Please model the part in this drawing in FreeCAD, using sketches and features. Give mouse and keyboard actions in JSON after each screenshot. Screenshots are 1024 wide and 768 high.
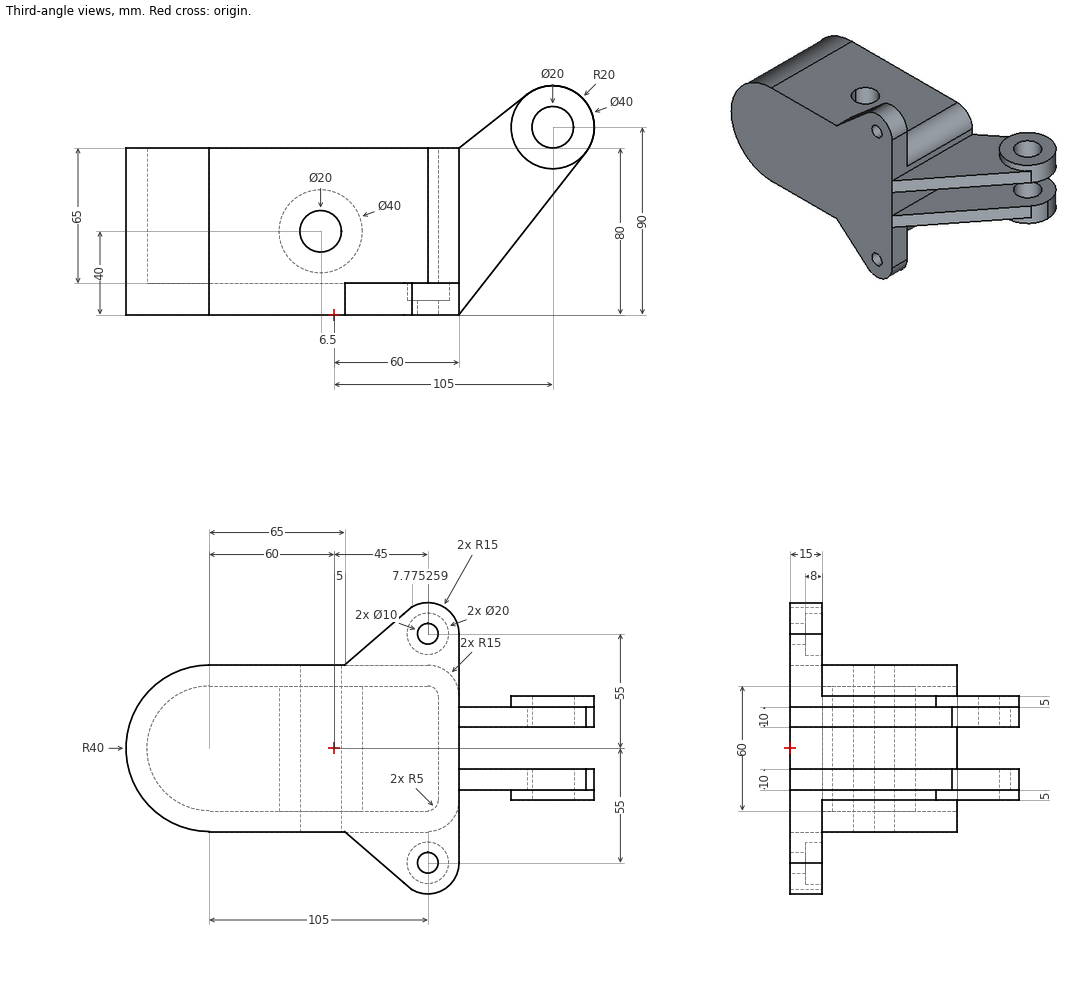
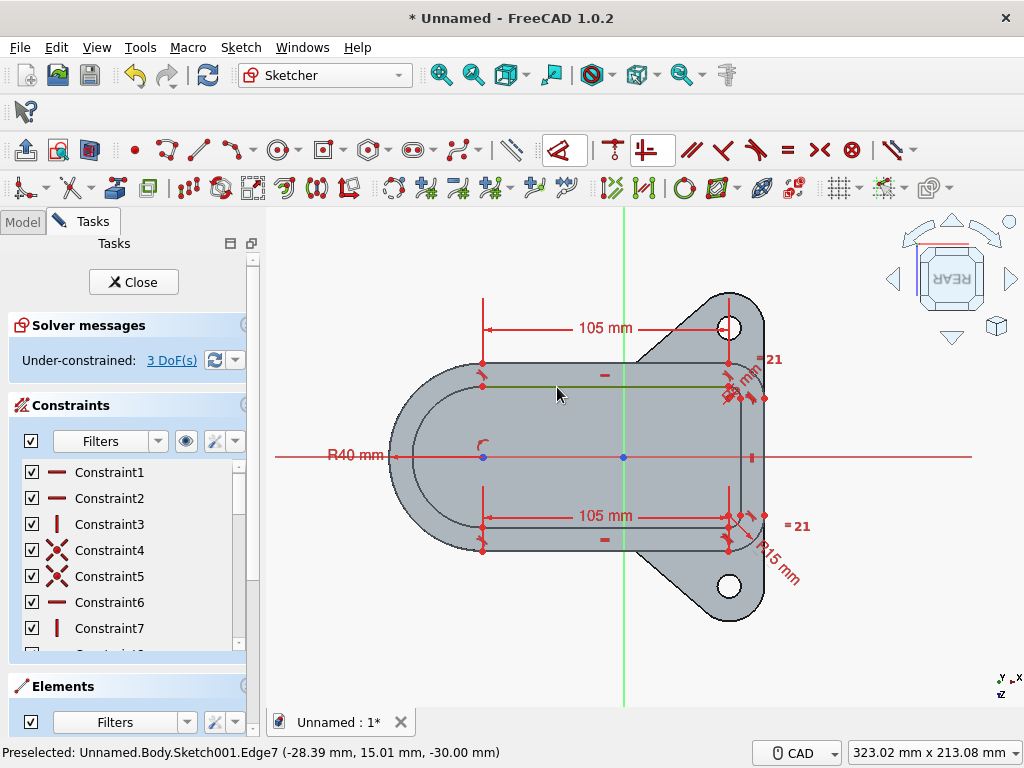
{"action": "key", "text": "l"}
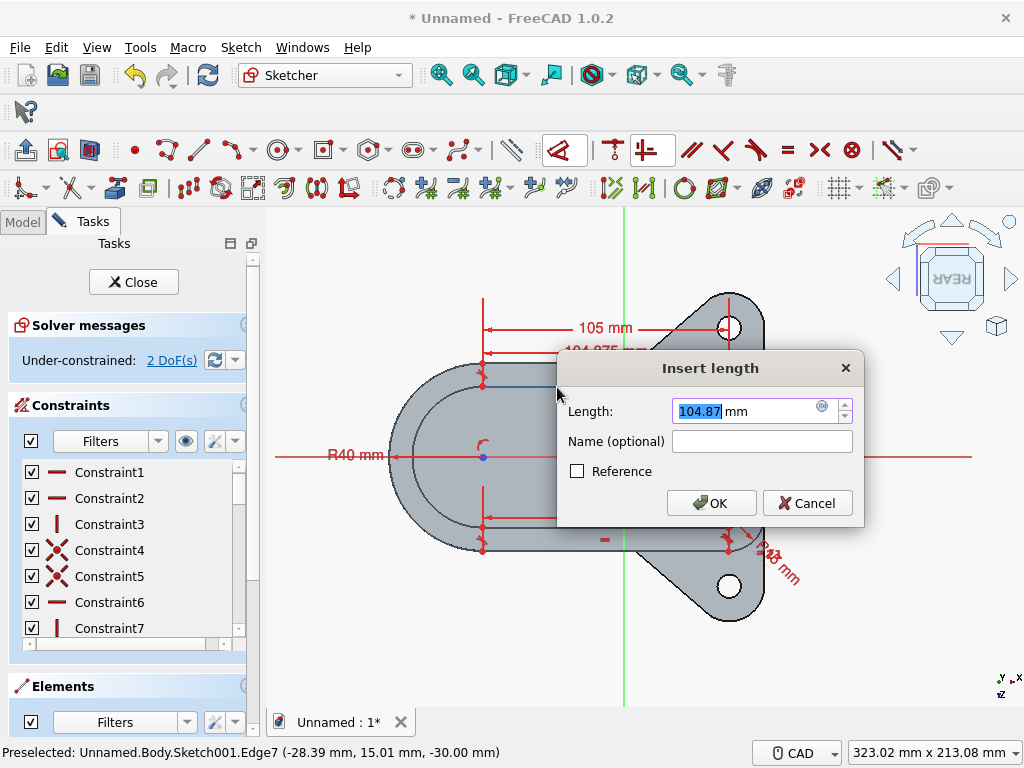
{"action": "type", "text": "105"}
{"action": "key", "text": "Return"}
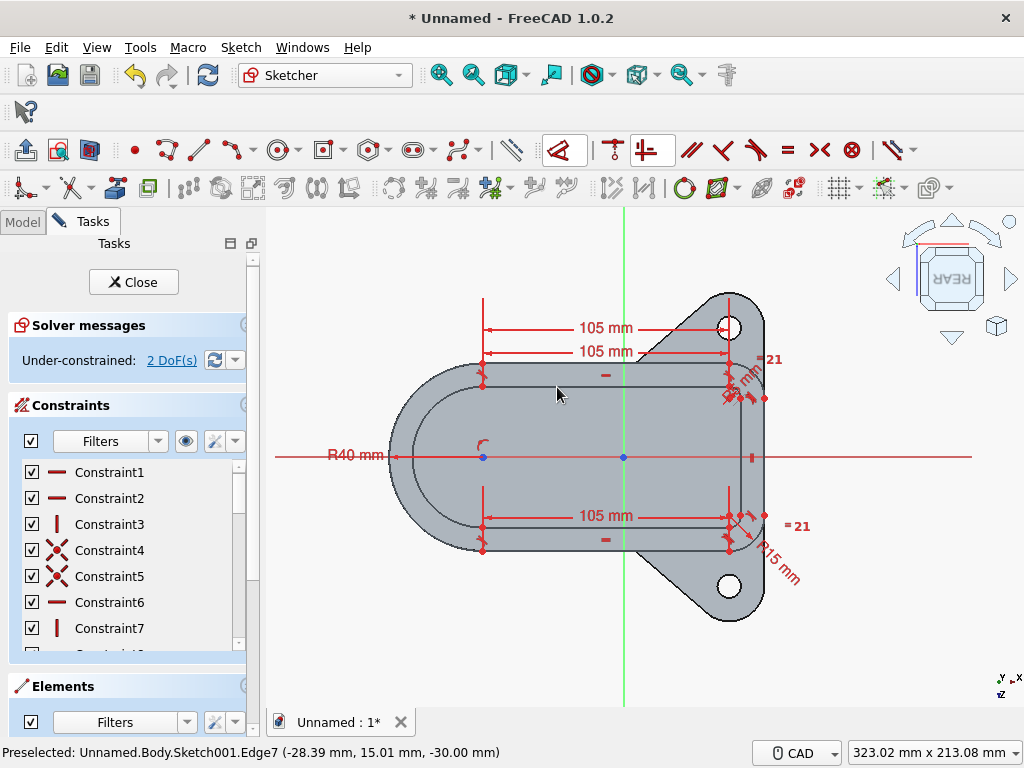
{"action": "left_click", "coordinate": [729, 363]}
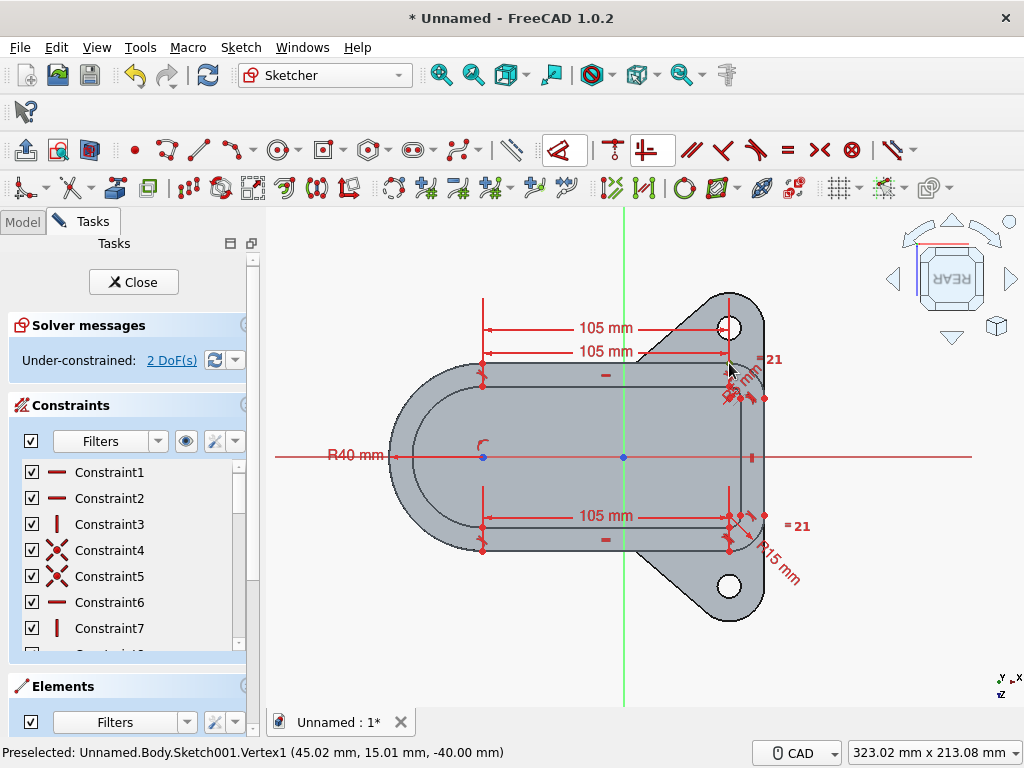
{"action": "left_click", "coordinate": [582, 150]}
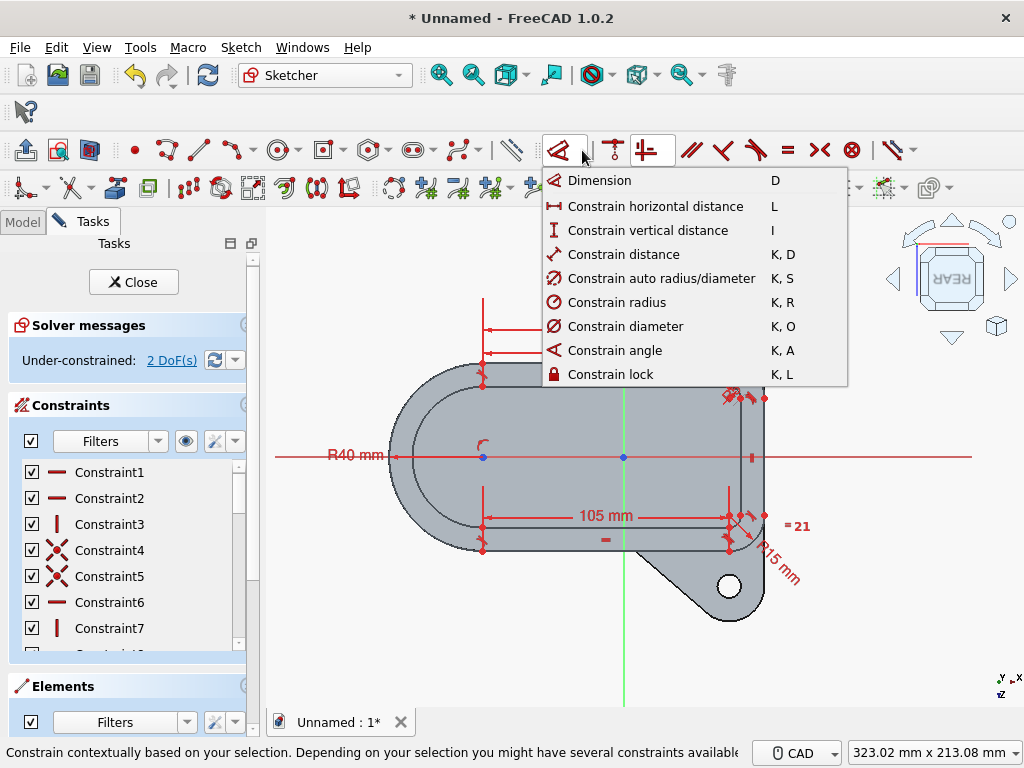
{"action": "left_click", "coordinate": [695, 206]}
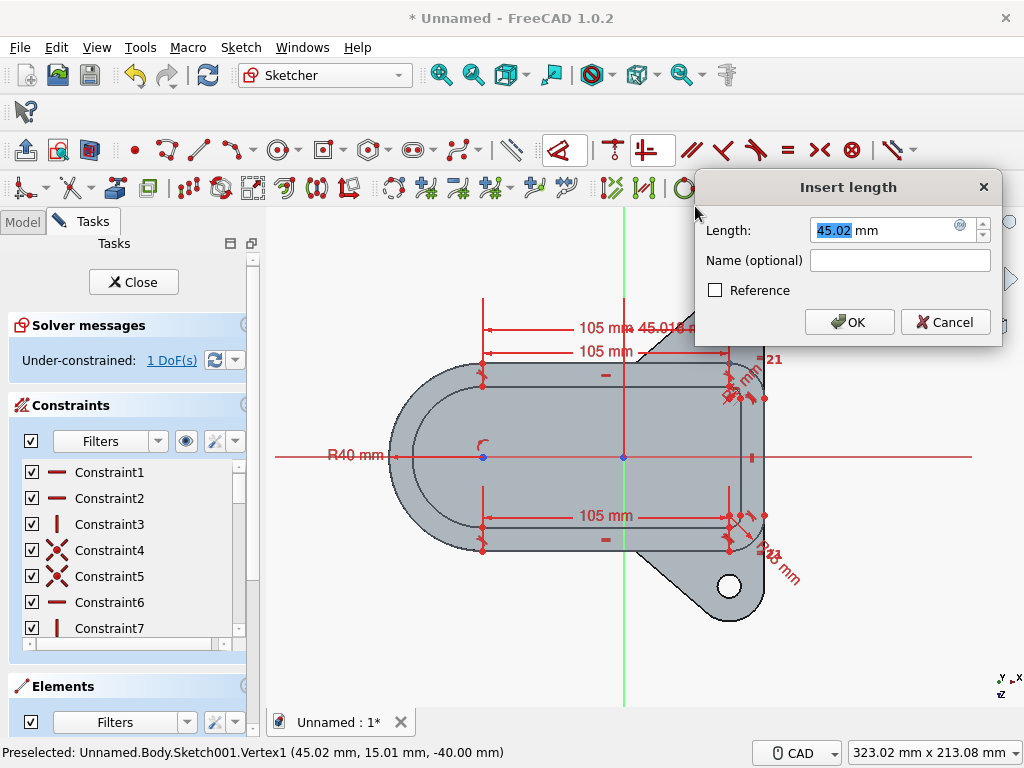
{"action": "type", "text": "45"}
{"action": "key", "text": "Return"}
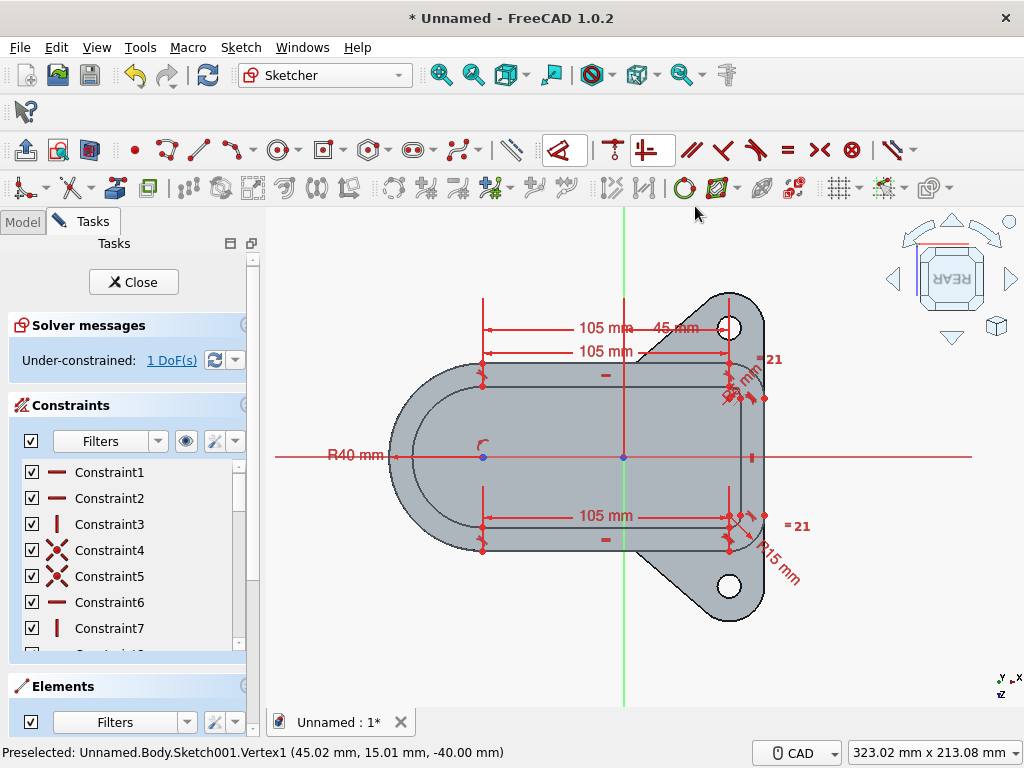
{"action": "left_click", "coordinate": [483, 457]}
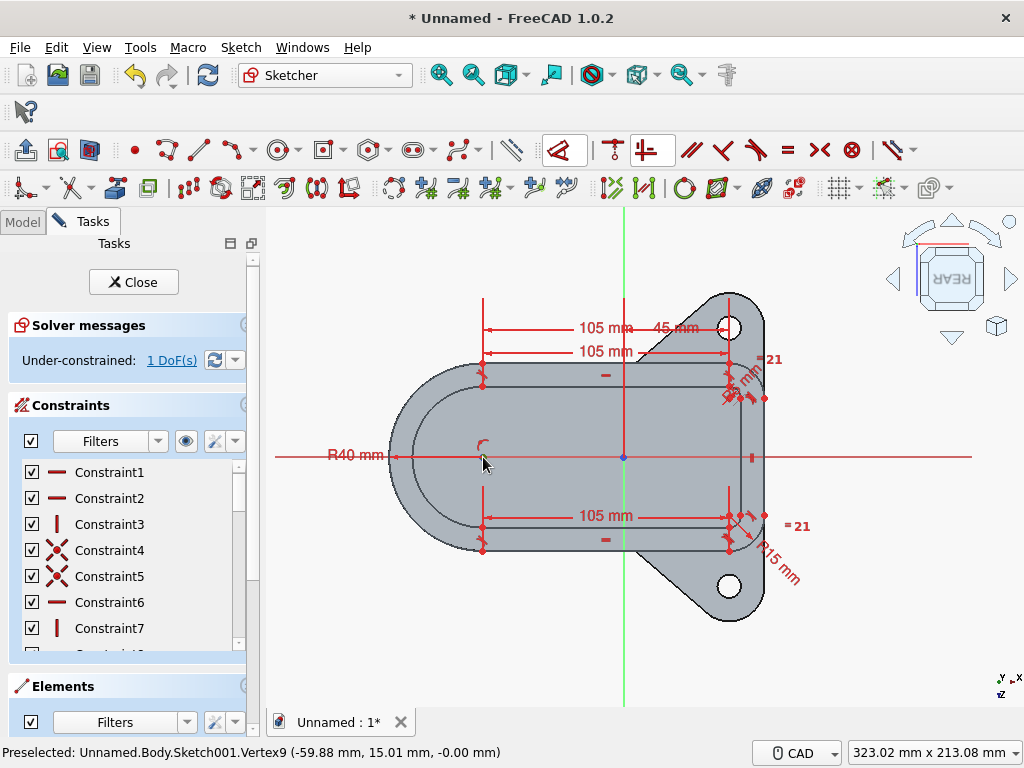
{"action": "key", "text": "l"}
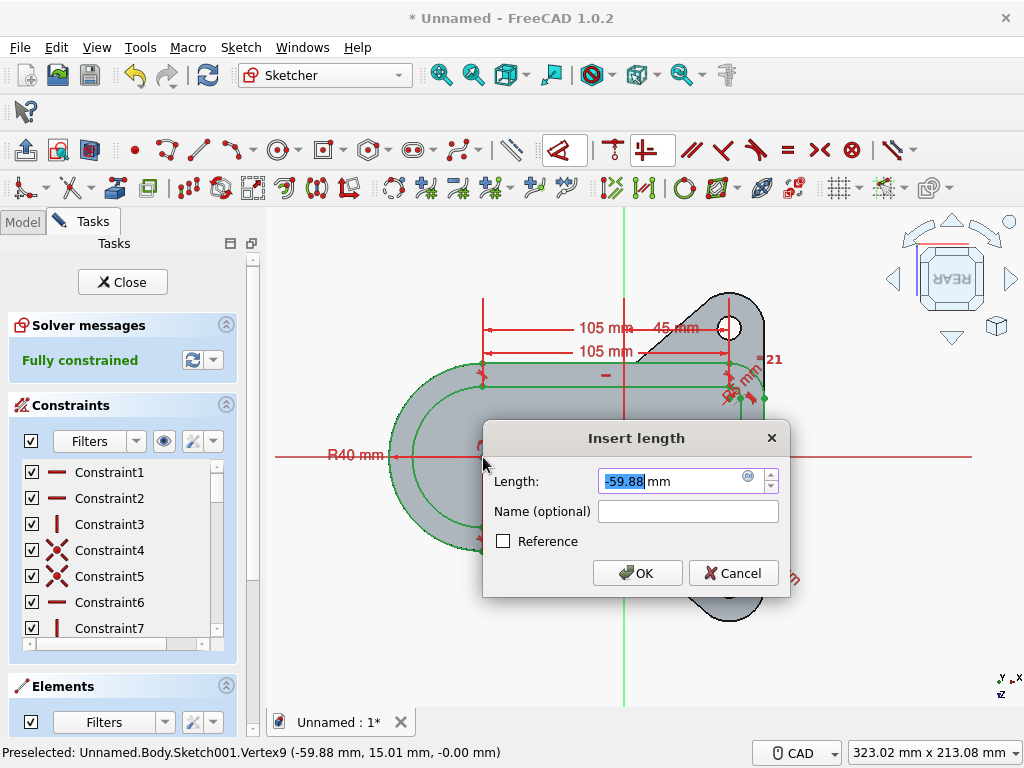
{"action": "type", "text": "-60"}
{"action": "key", "text": "Return"}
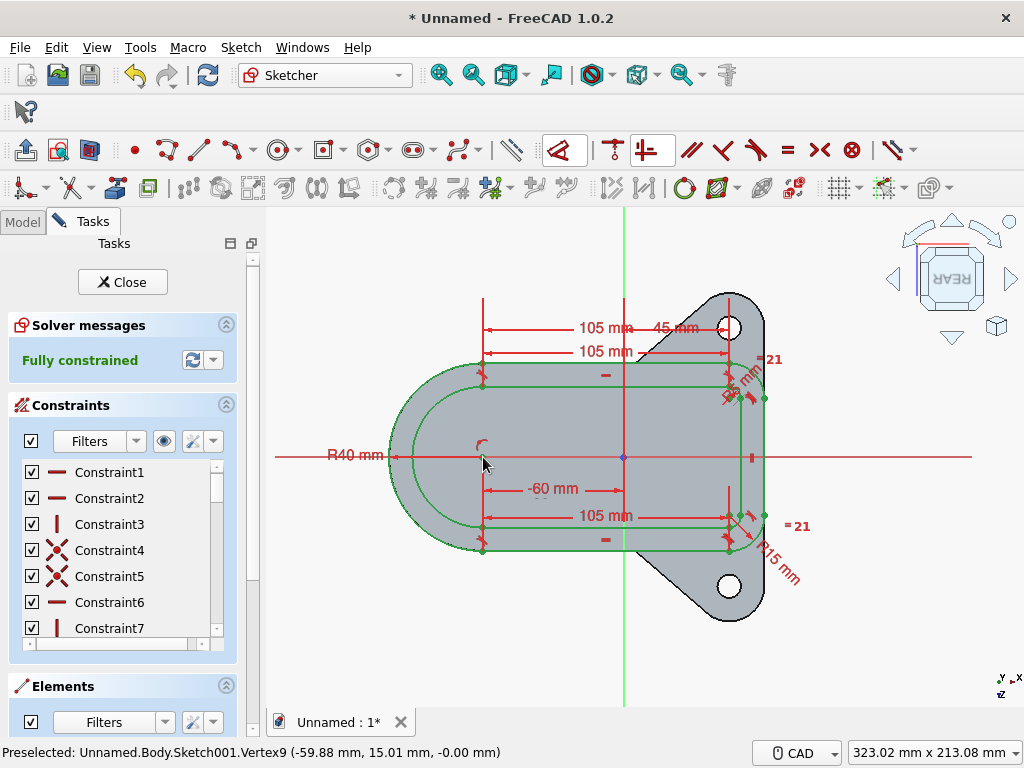
{"action": "left_click", "coordinate": [123, 282]}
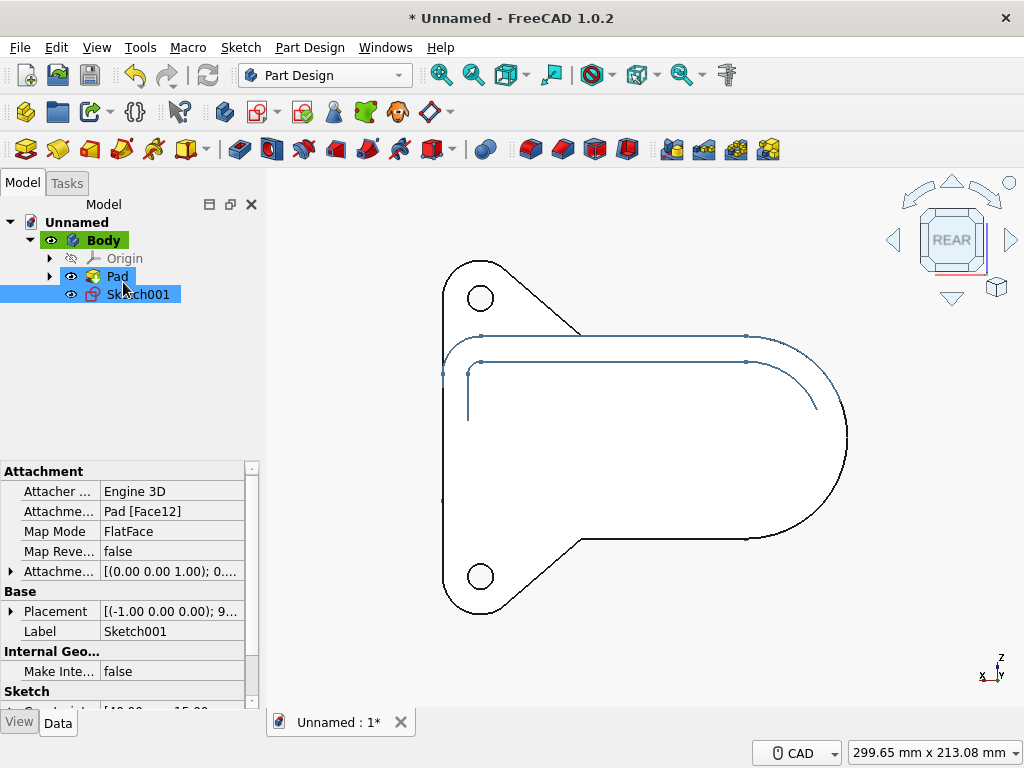
{"action": "left_click", "coordinate": [26, 150]}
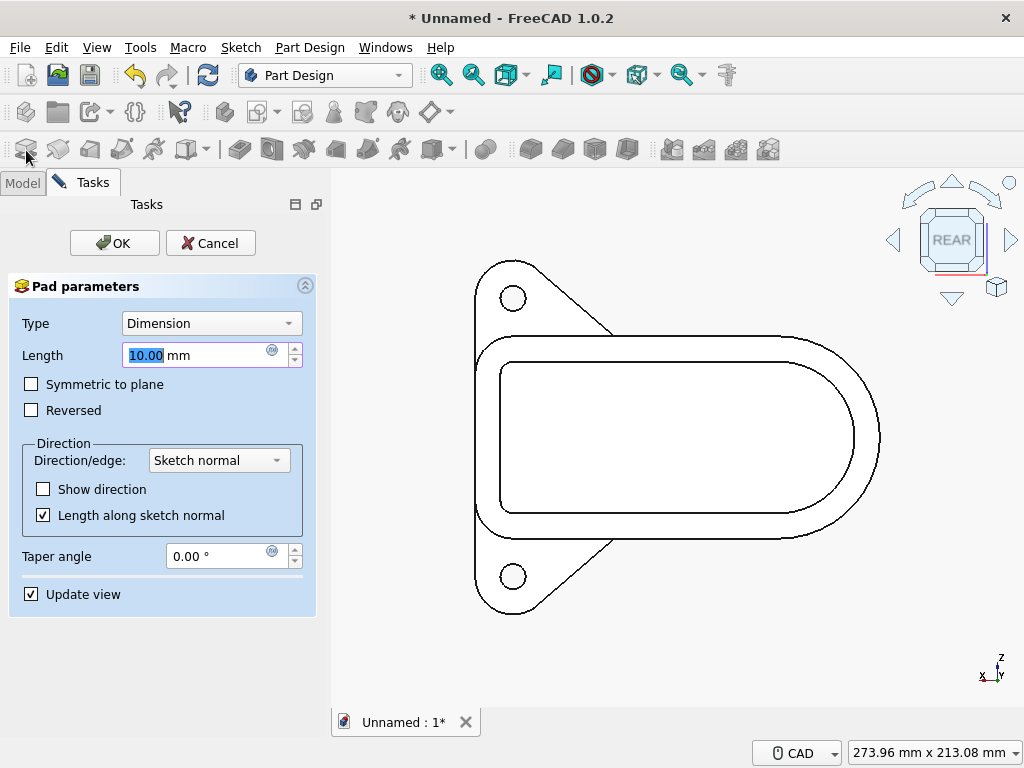
{"action": "type", "text": "65"}
{"action": "key", "text": "Tab"}